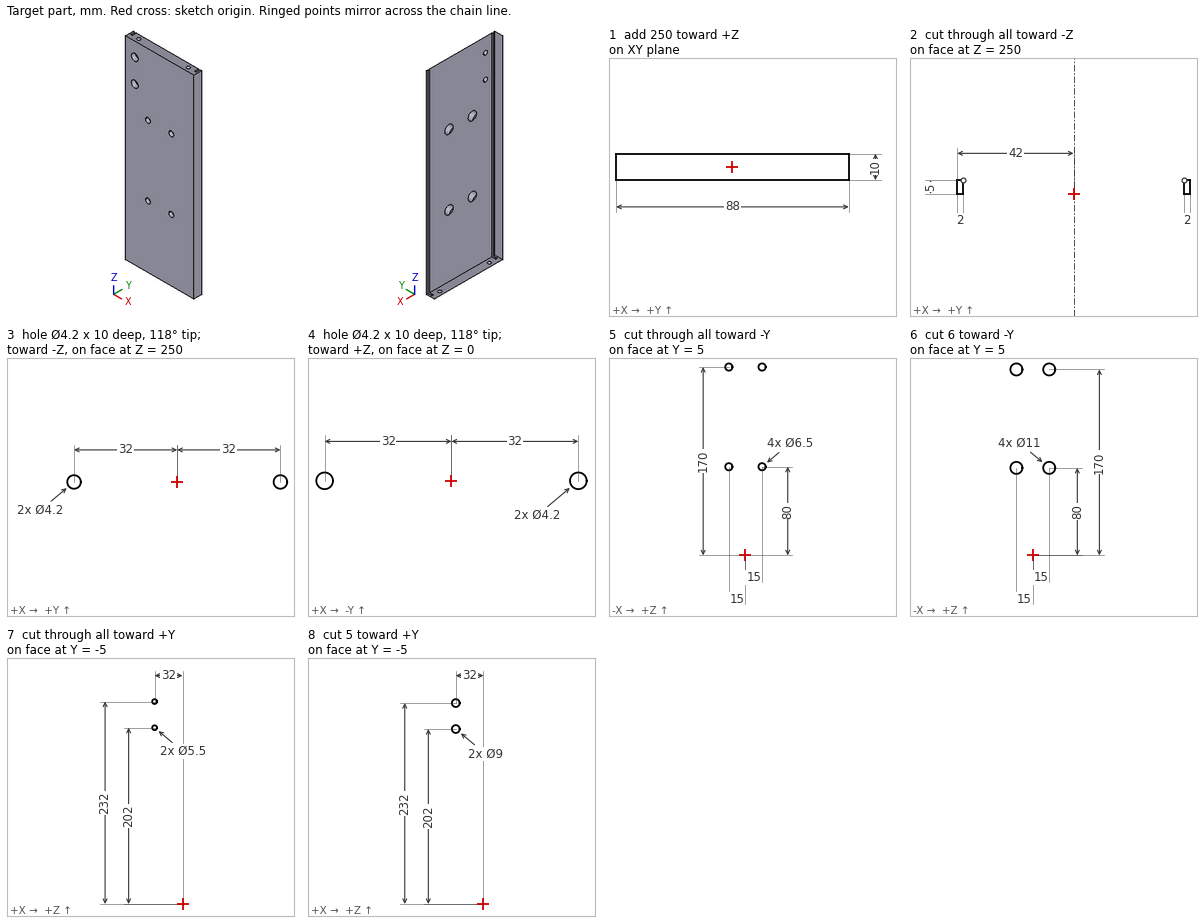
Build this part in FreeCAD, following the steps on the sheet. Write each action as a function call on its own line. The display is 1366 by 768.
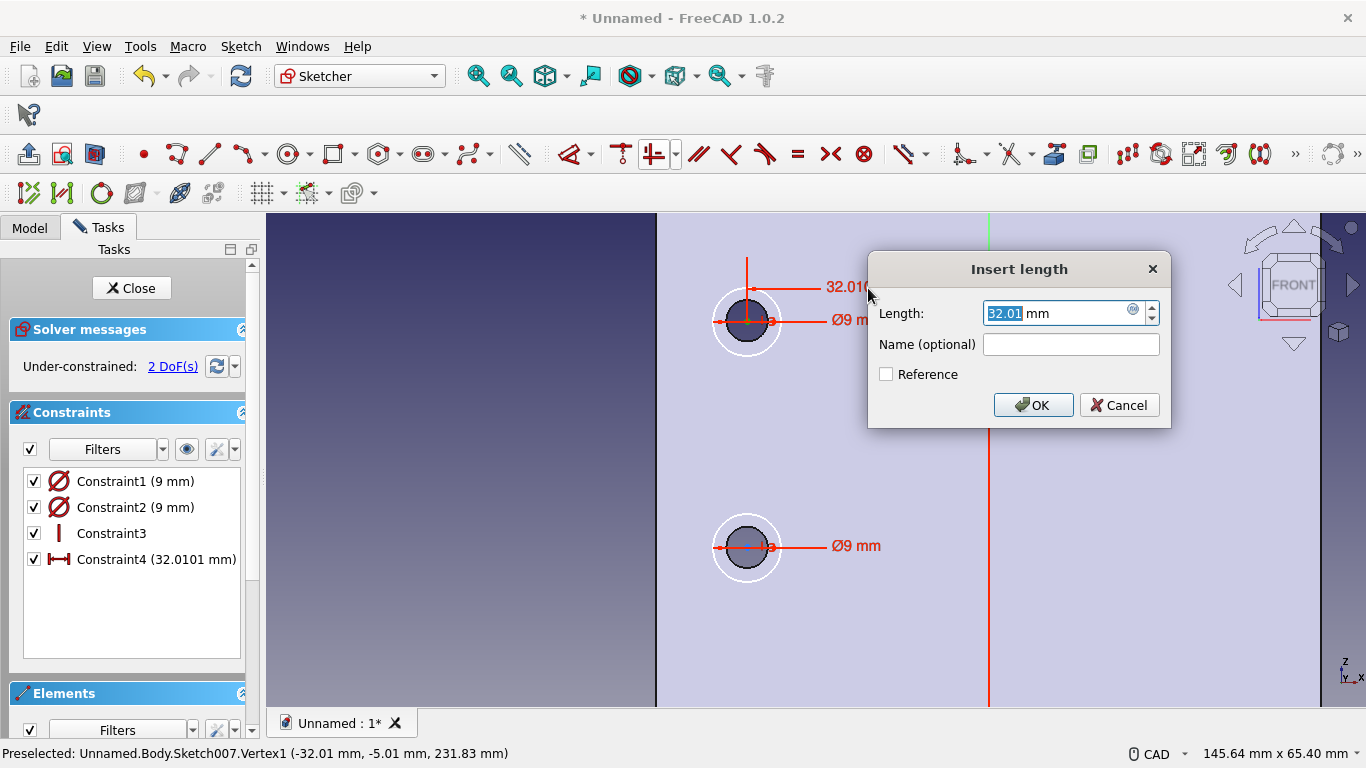
text(32)
key(Return)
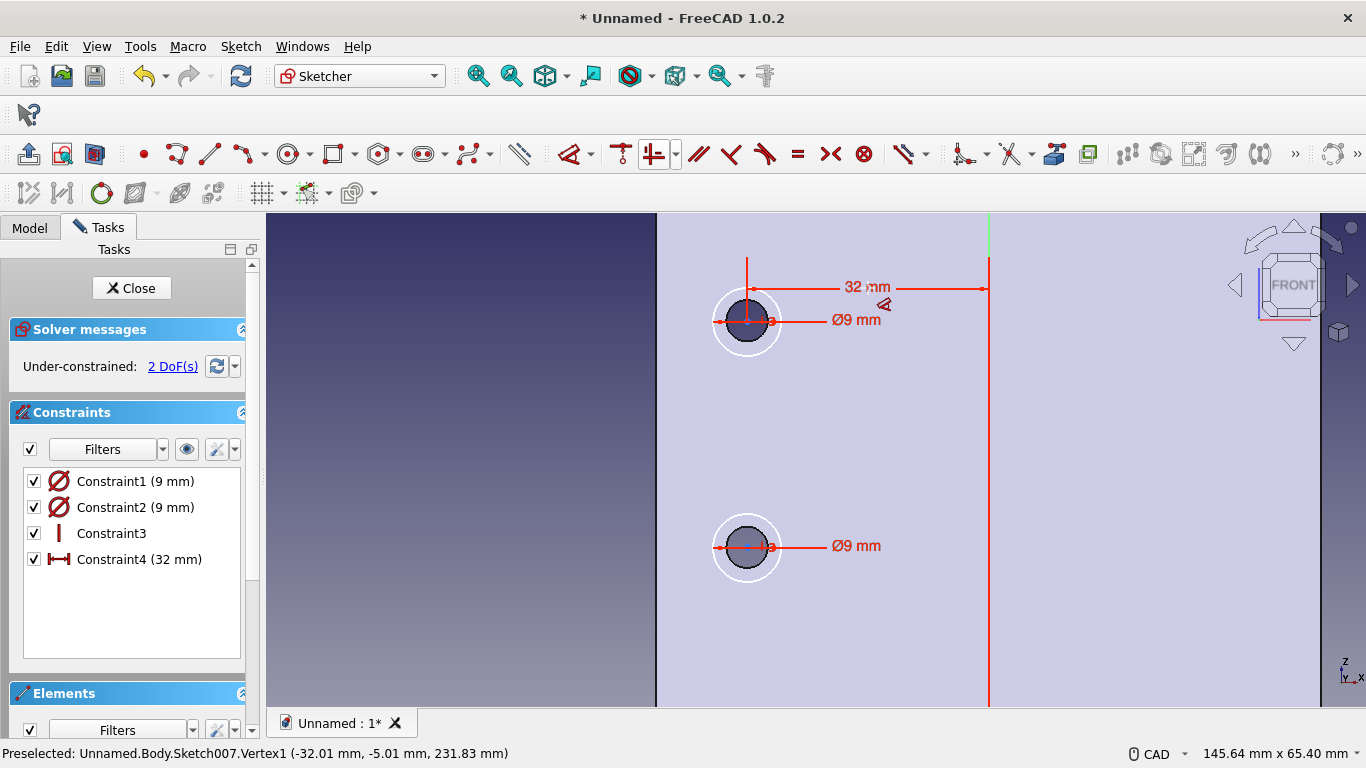
click(747, 322)
click(1023, 500)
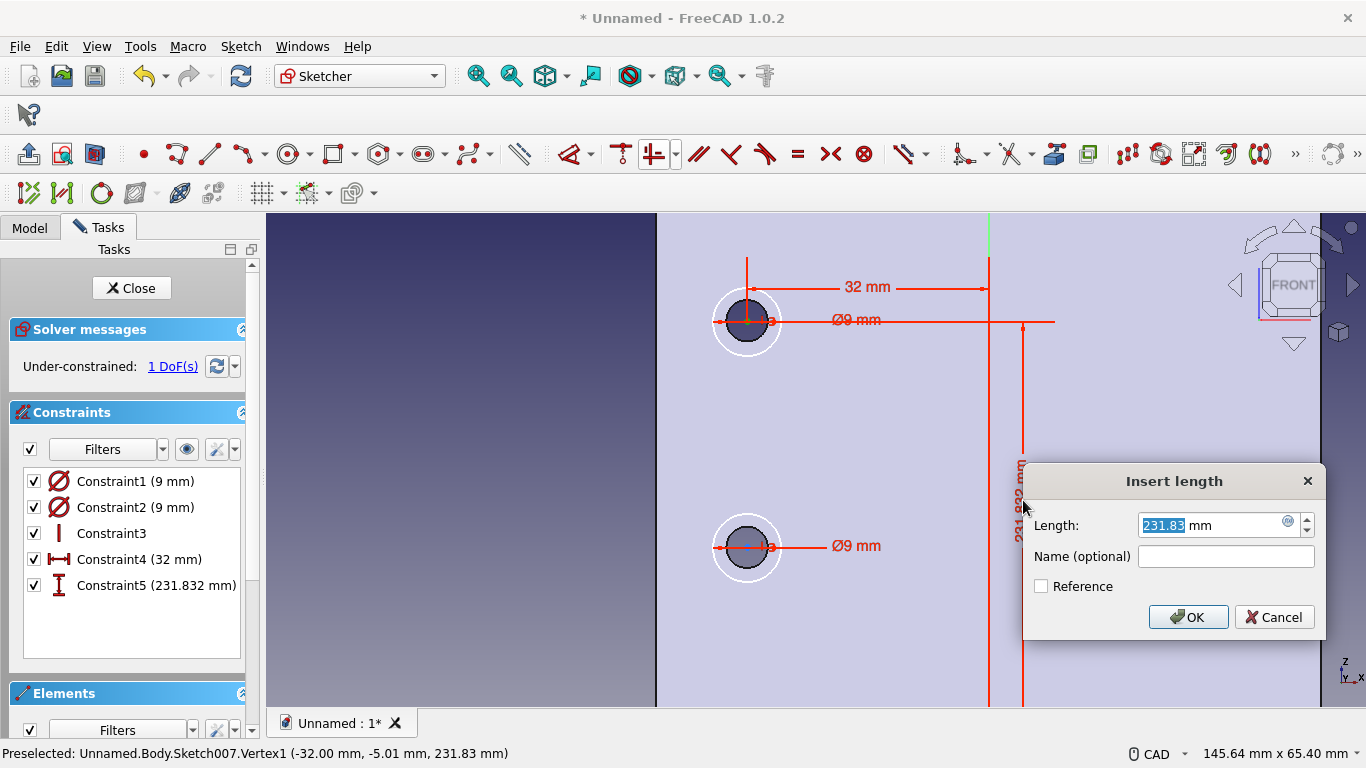
text(232)
key(Return)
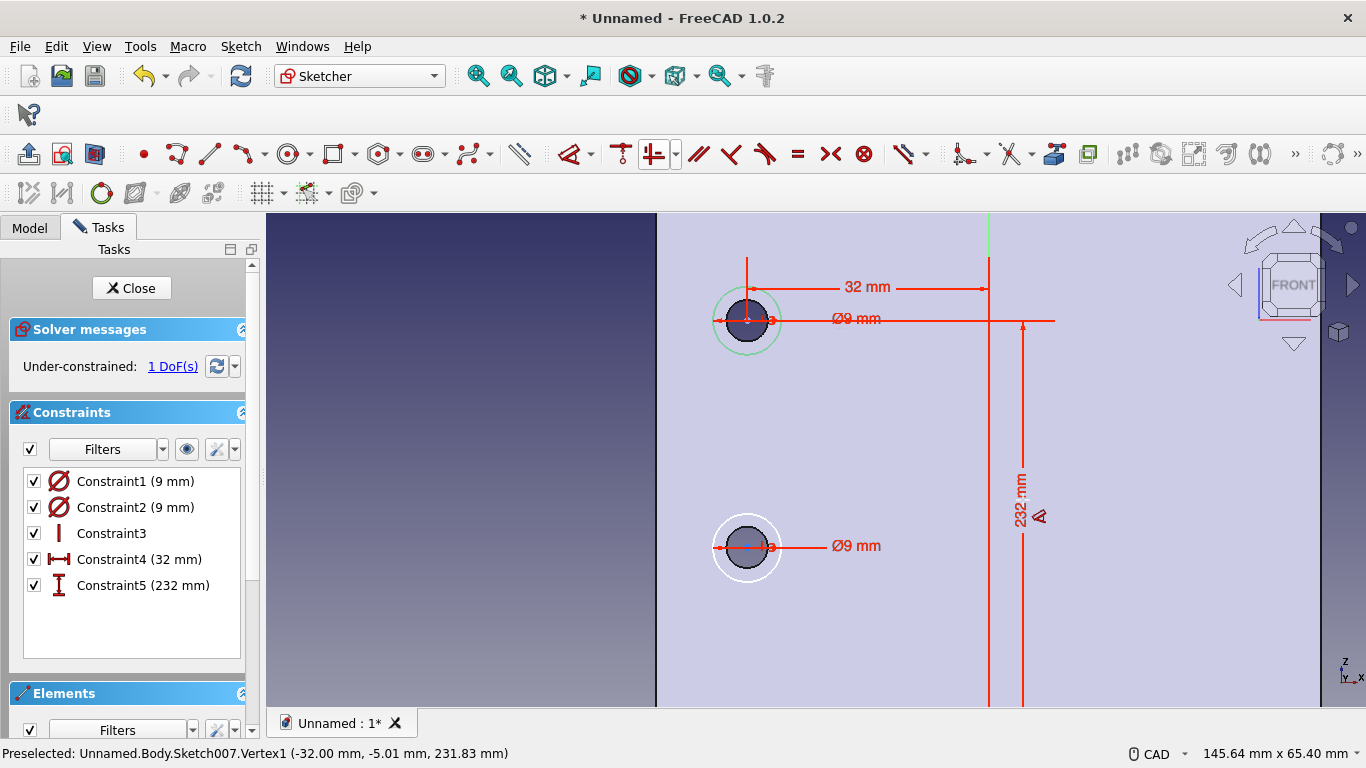
click(747, 548)
click(1023, 613)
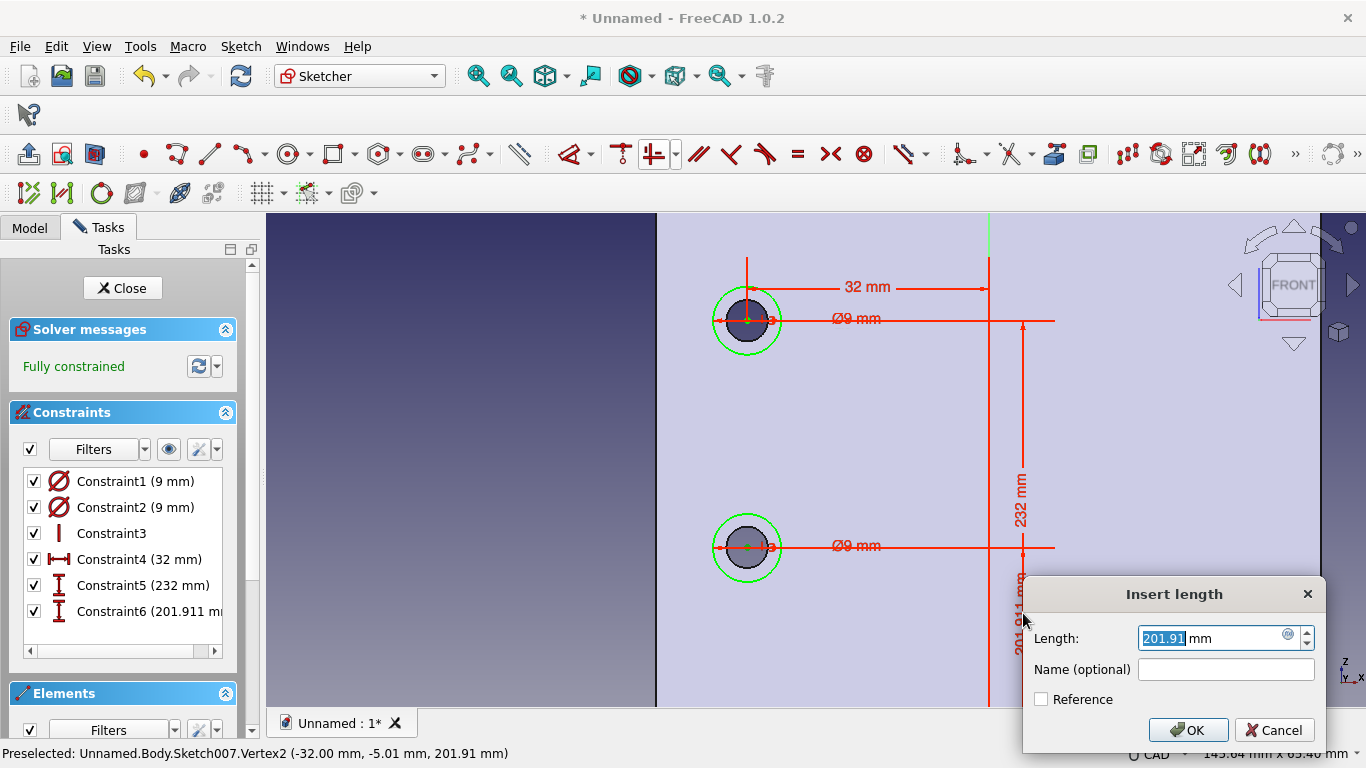
text(202)
key(Return)
key(Escape)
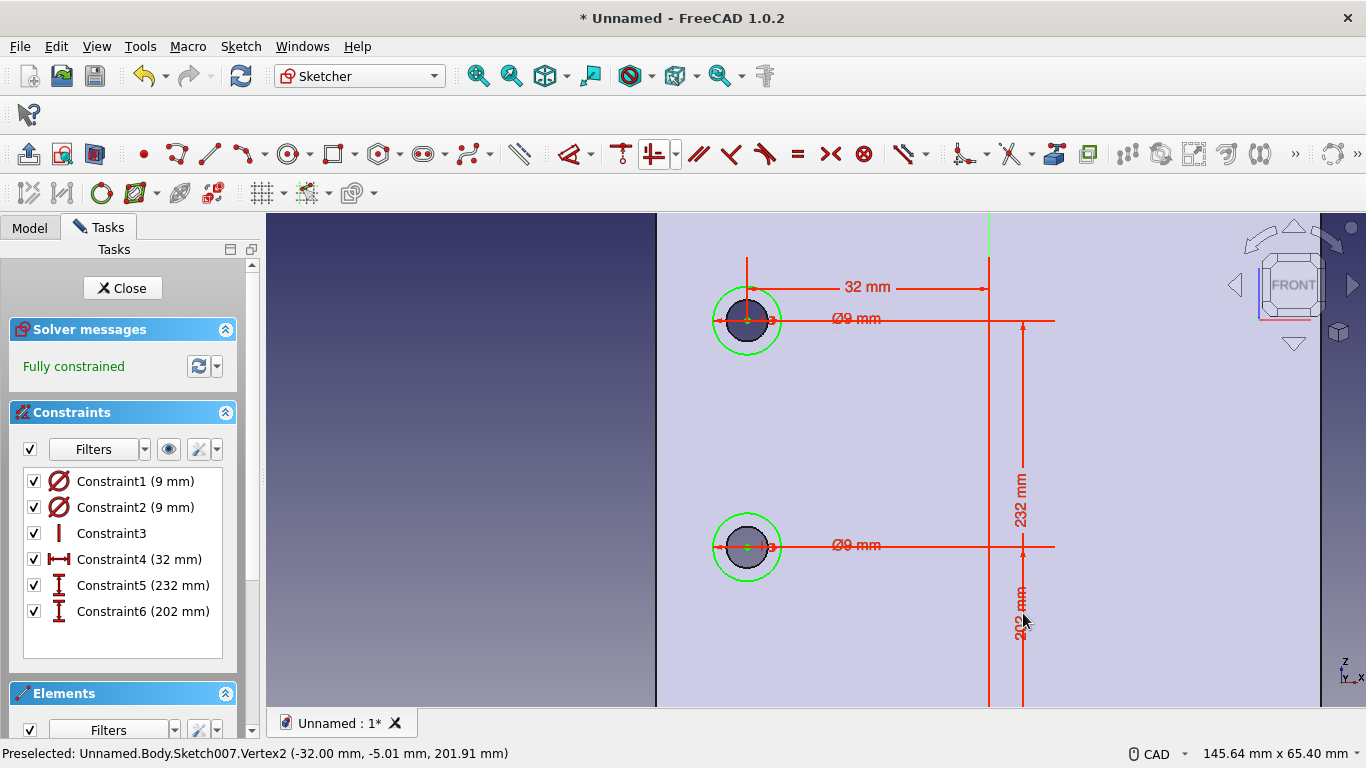
click(123, 288)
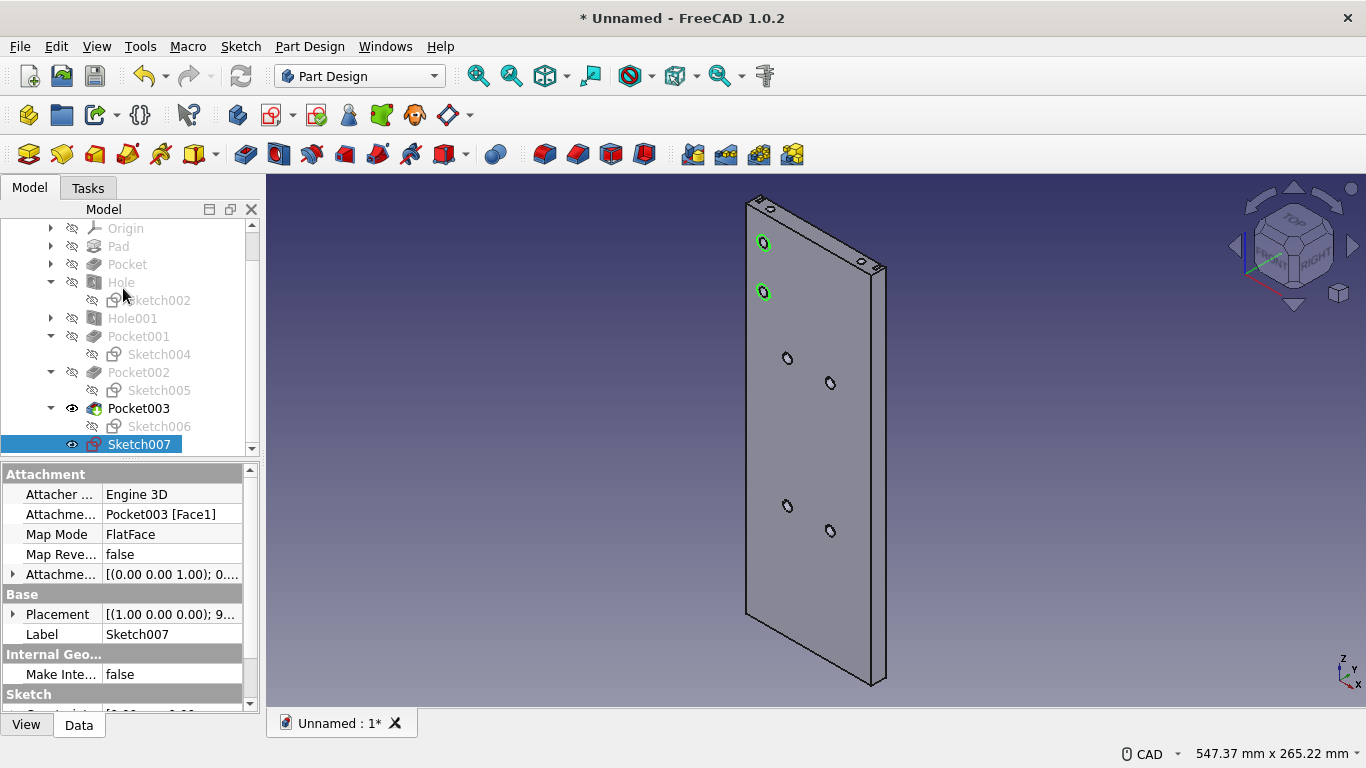
click(246, 154)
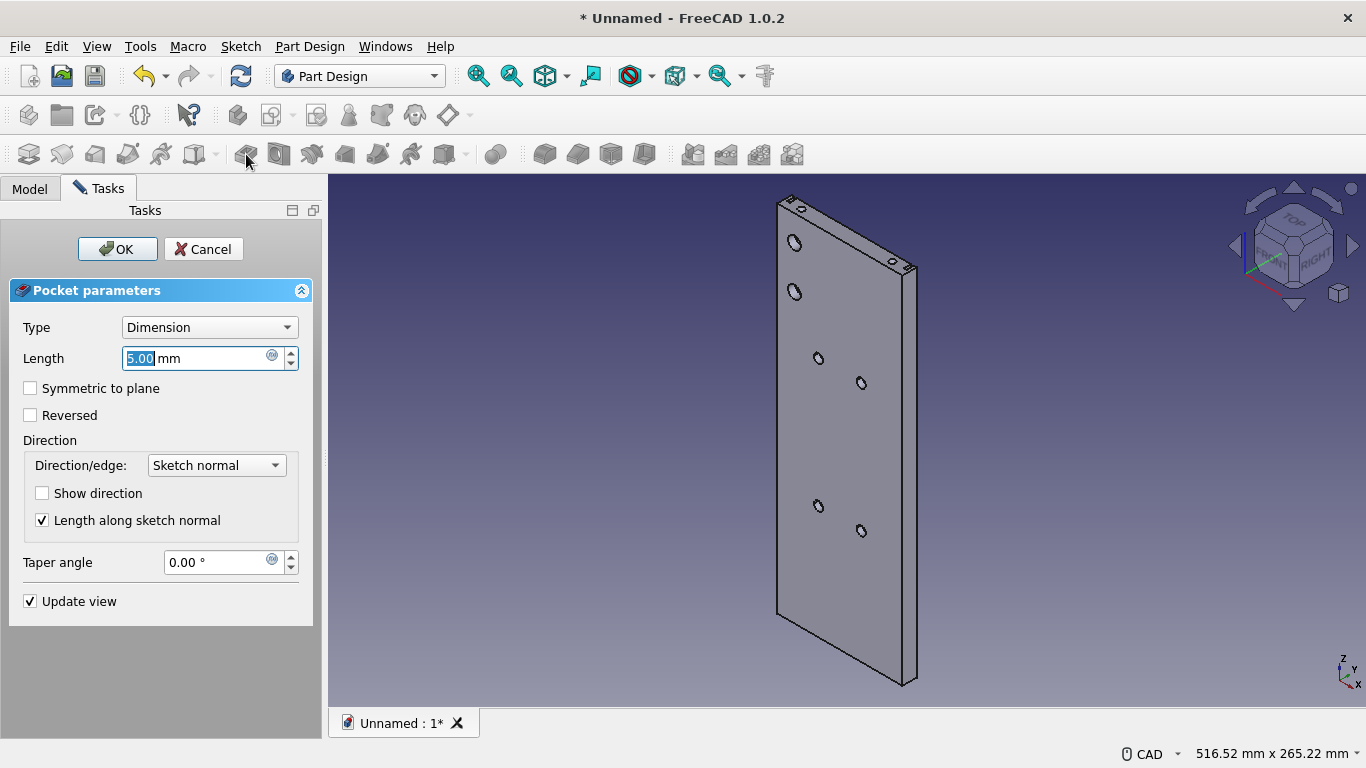
text(5)
key(Tab)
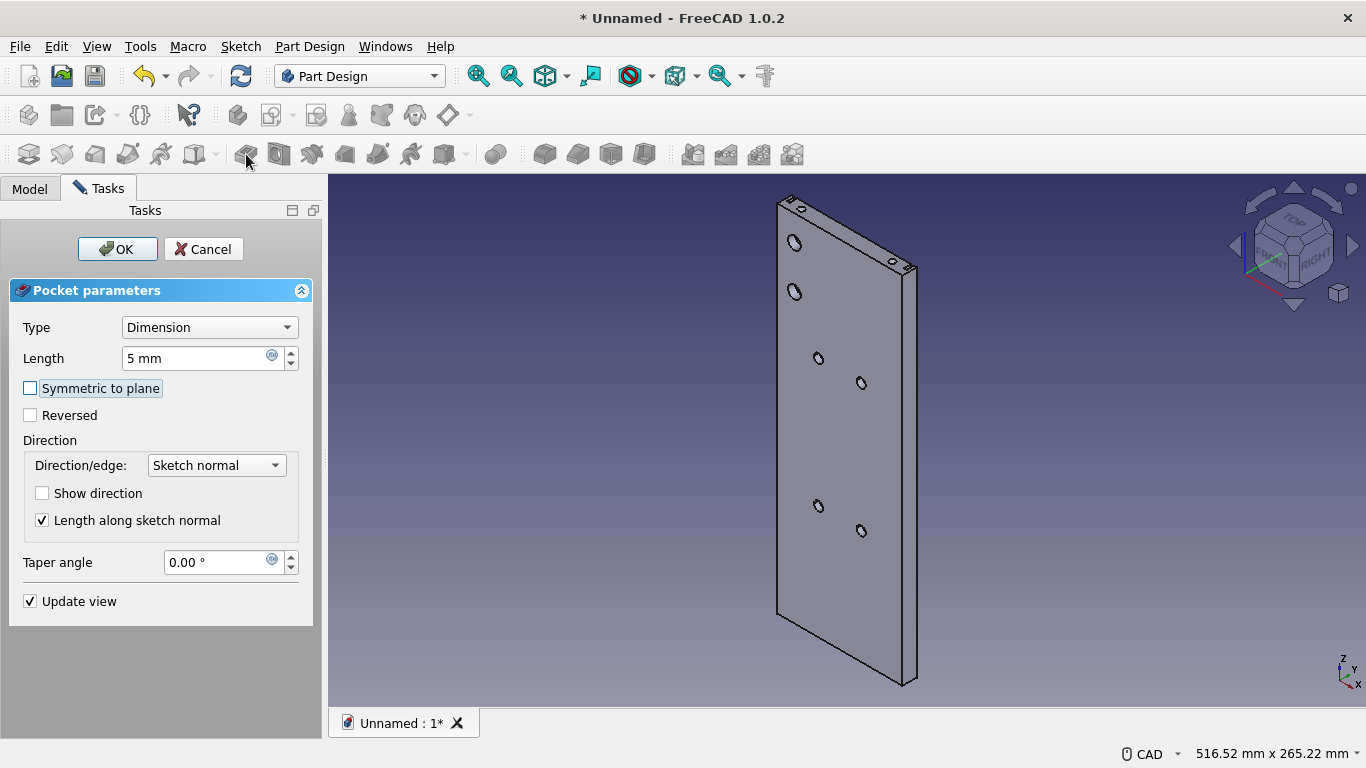
click(118, 249)